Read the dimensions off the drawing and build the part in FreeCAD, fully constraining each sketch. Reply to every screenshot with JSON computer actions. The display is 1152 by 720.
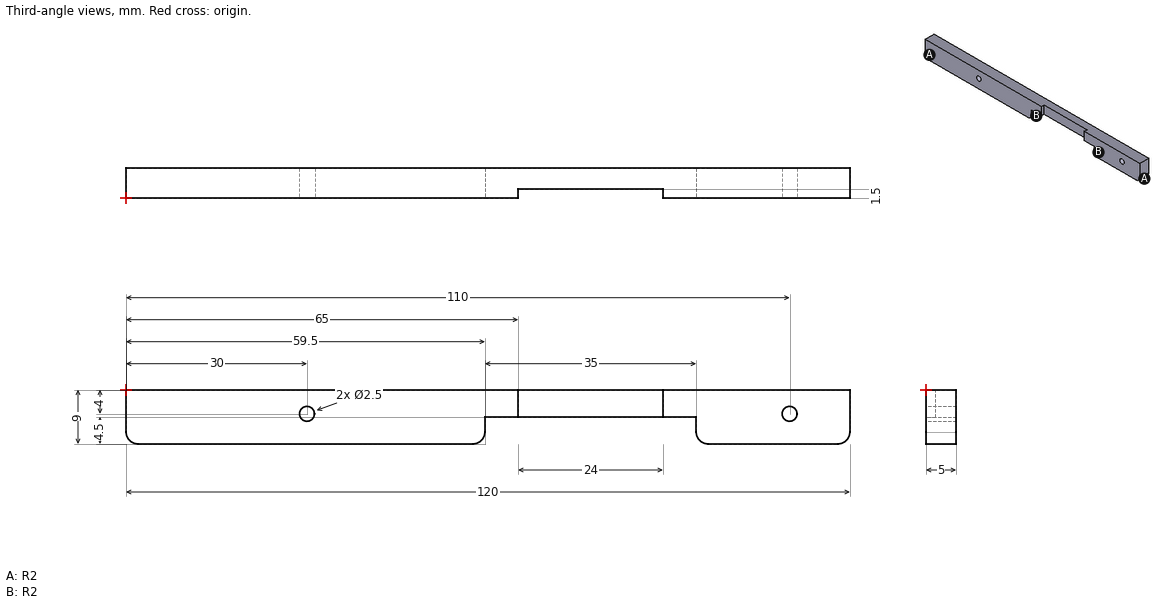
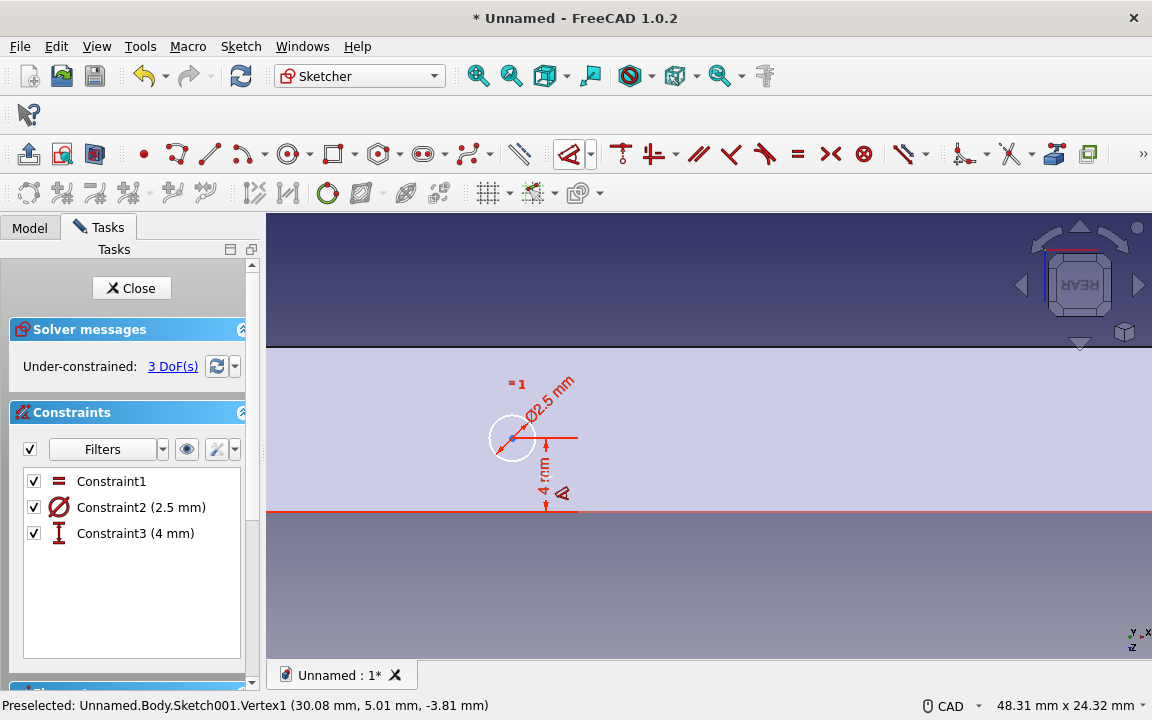
{"action": "scroll", "coordinate": [529, 427], "scroll_direction": "down", "scroll_amount": 7}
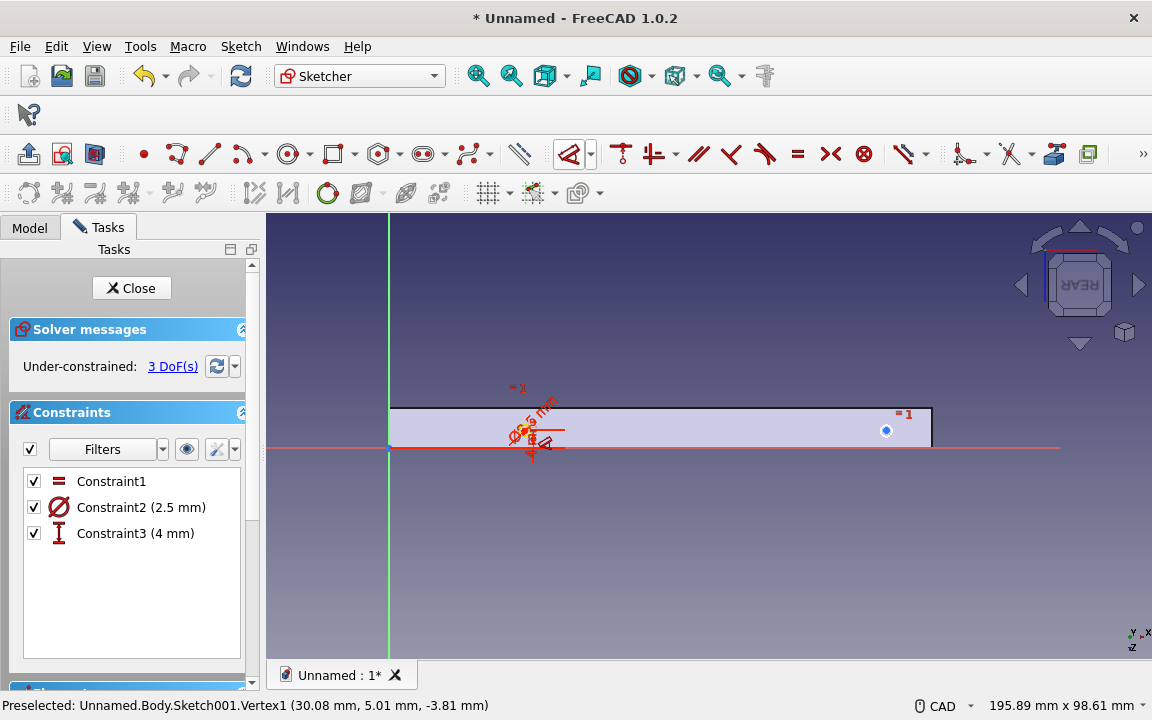
{"action": "scroll", "coordinate": [886, 431], "scroll_direction": "up", "scroll_amount": 4}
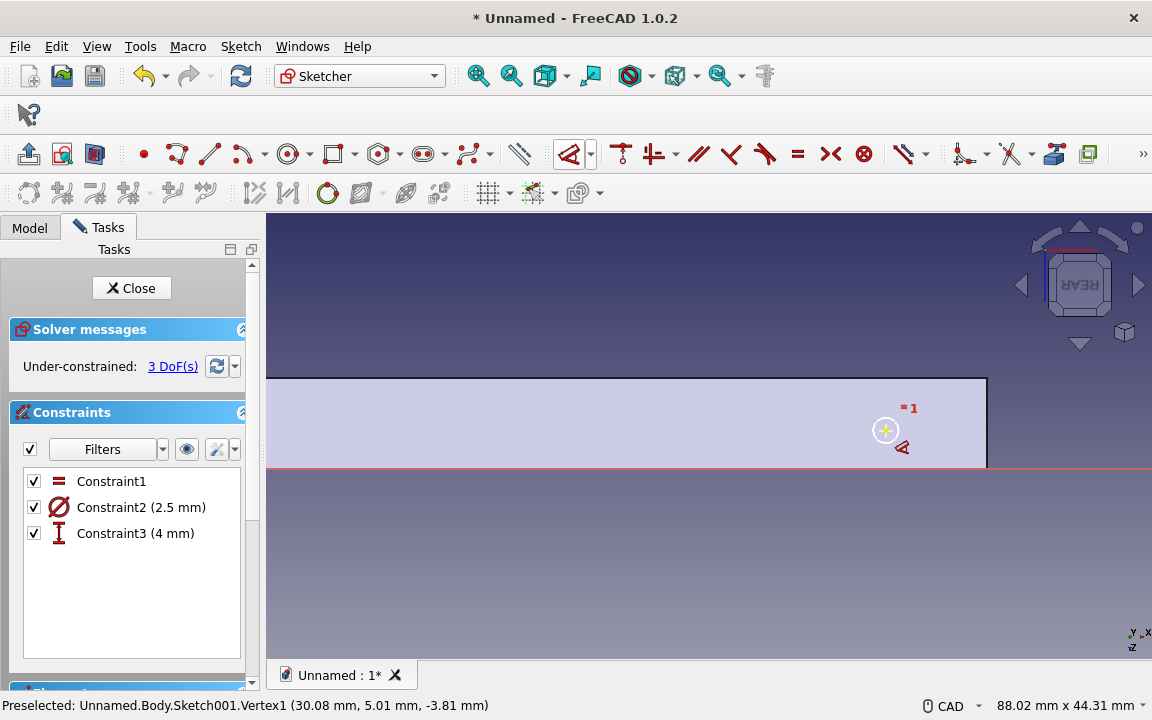
{"action": "left_click", "coordinate": [886, 430]}
{"action": "left_click", "coordinate": [920, 450]}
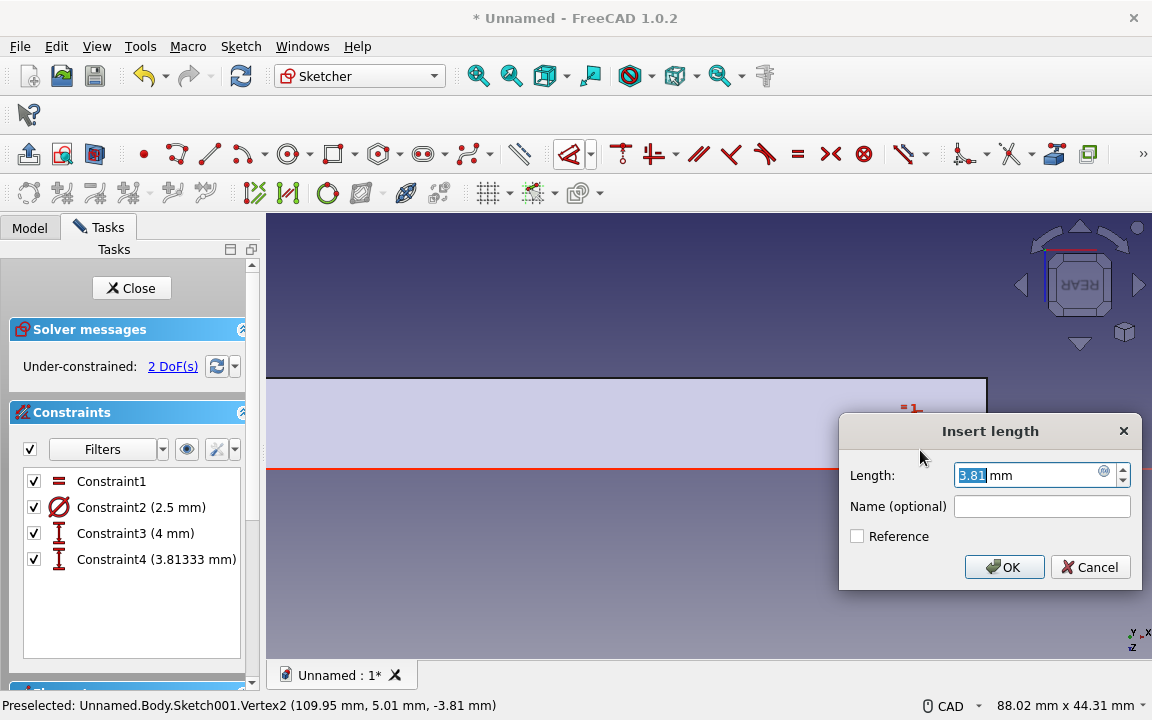
{"action": "type", "text": "4"}
{"action": "key", "text": "Return"}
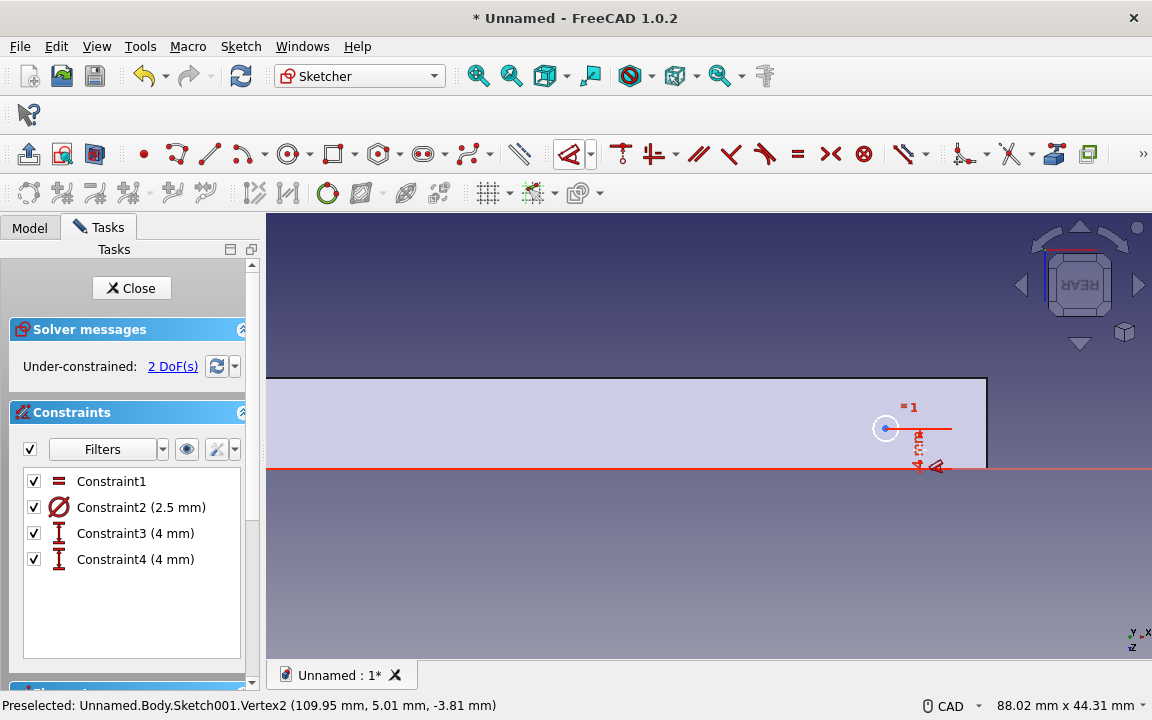
{"action": "scroll", "coordinate": [886, 431], "scroll_direction": "down", "scroll_amount": 4}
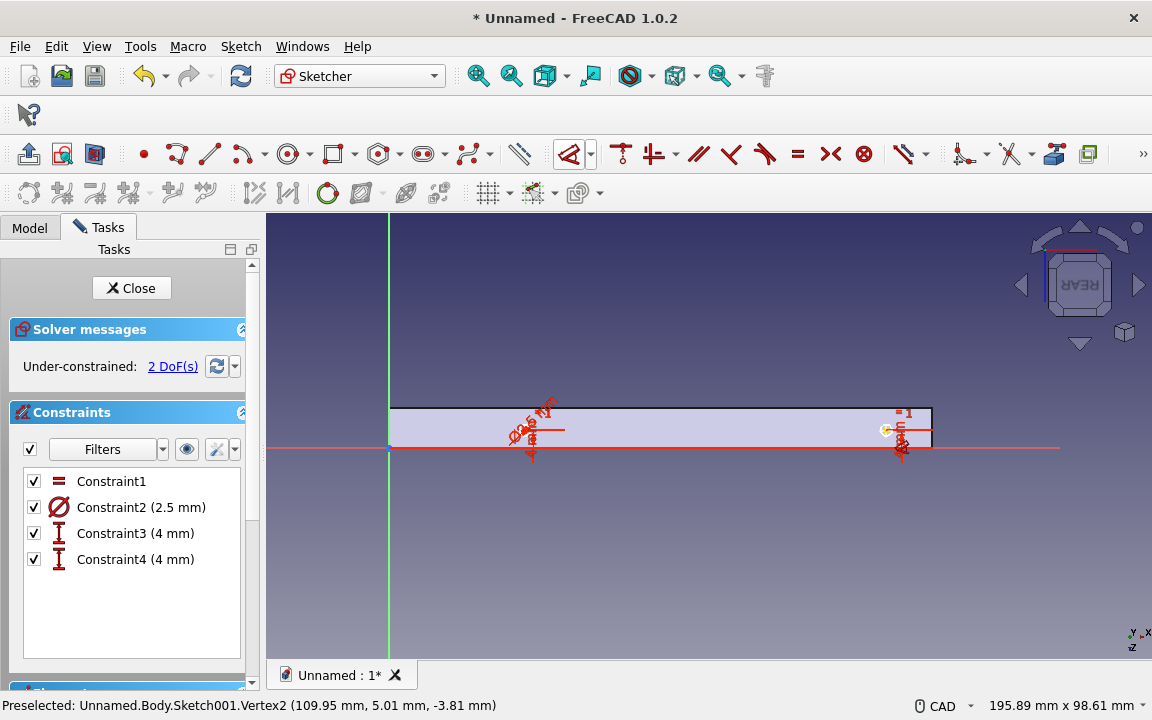
{"action": "left_click", "coordinate": [525, 430]}
{"action": "left_click", "coordinate": [457, 482]}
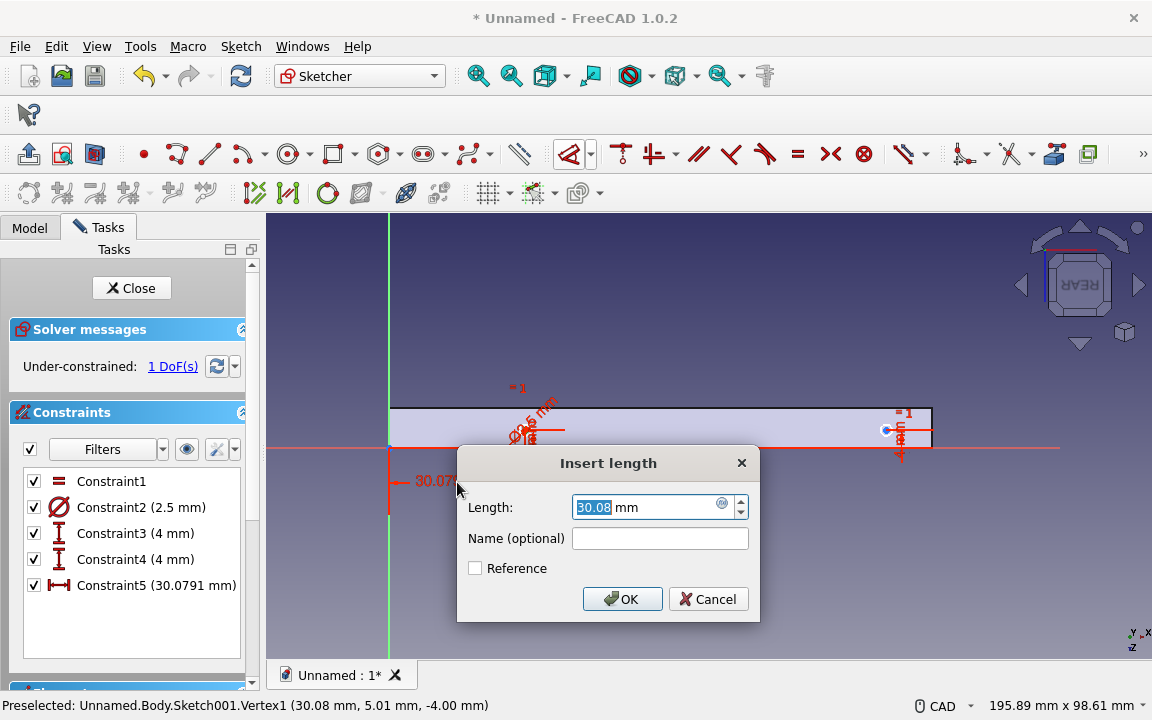
{"action": "type", "text": "30"}
{"action": "key", "text": "Return"}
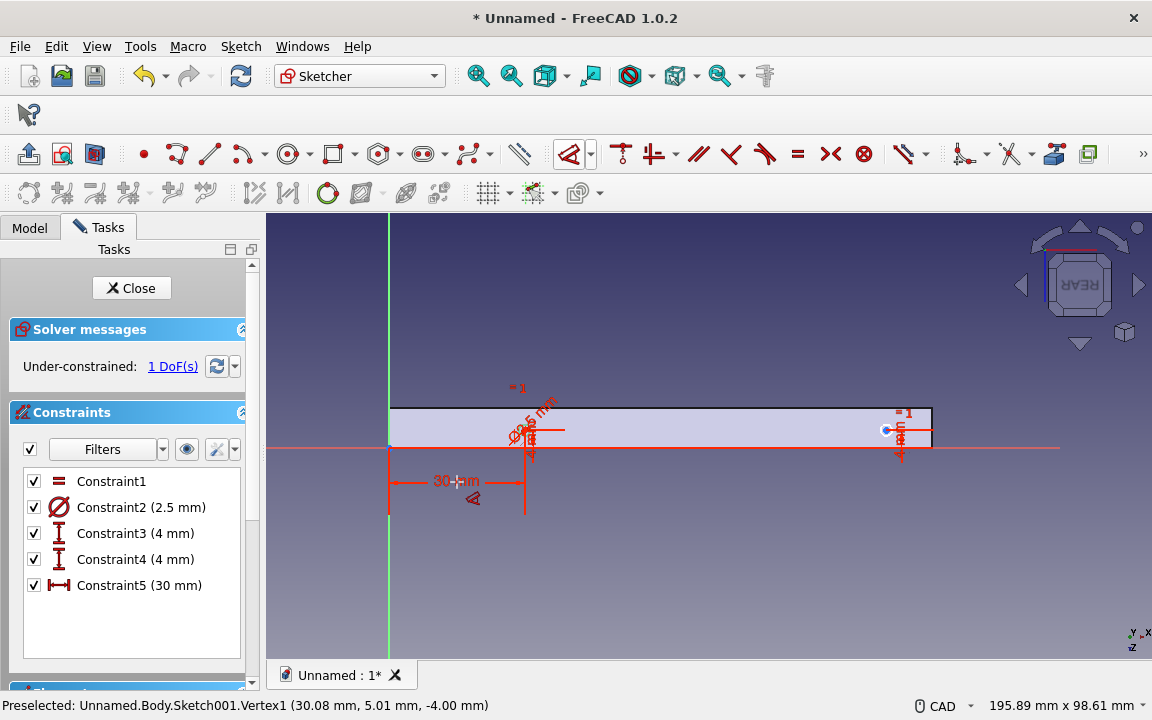
{"action": "left_click", "coordinate": [886, 430]}
{"action": "left_click", "coordinate": [638, 482]}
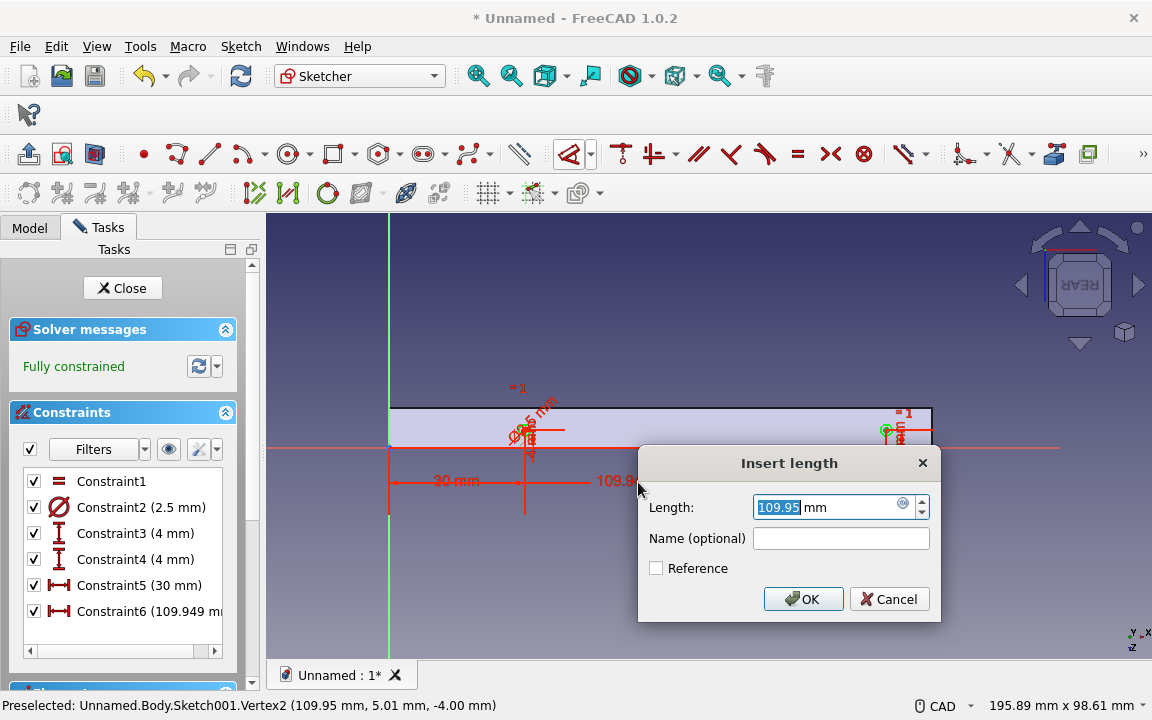
{"action": "type", "text": "110"}
{"action": "key", "text": "Return"}
{"action": "key", "text": "Escape"}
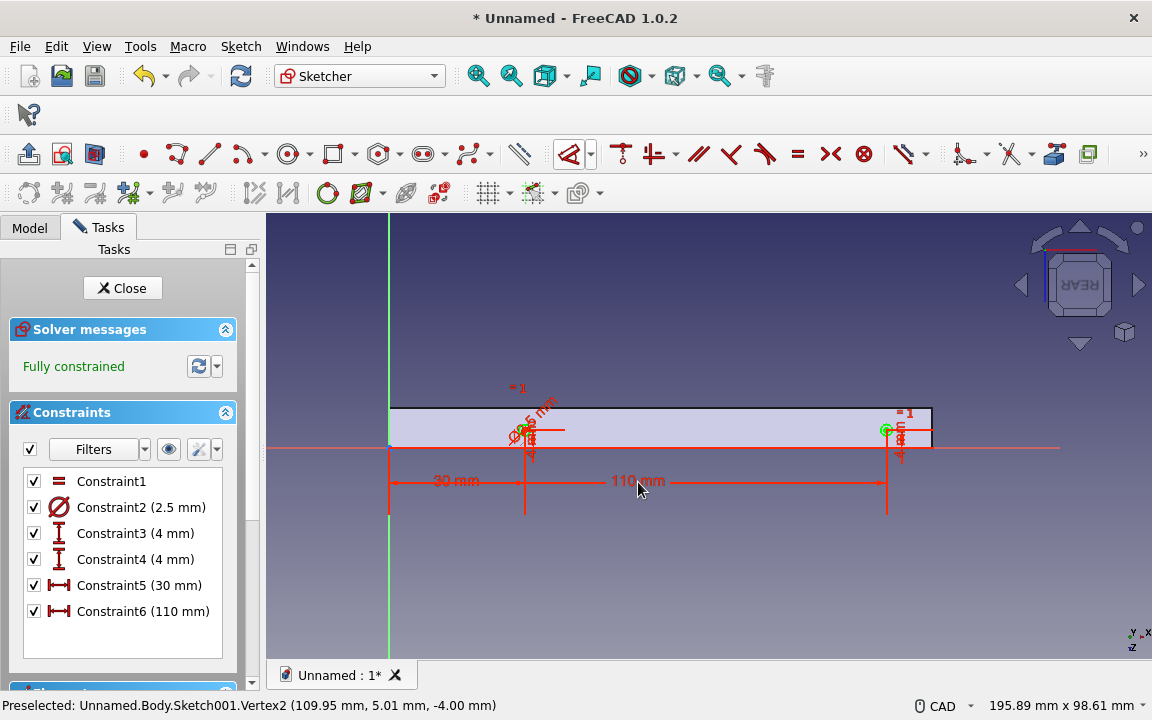
{"action": "left_click", "coordinate": [123, 288]}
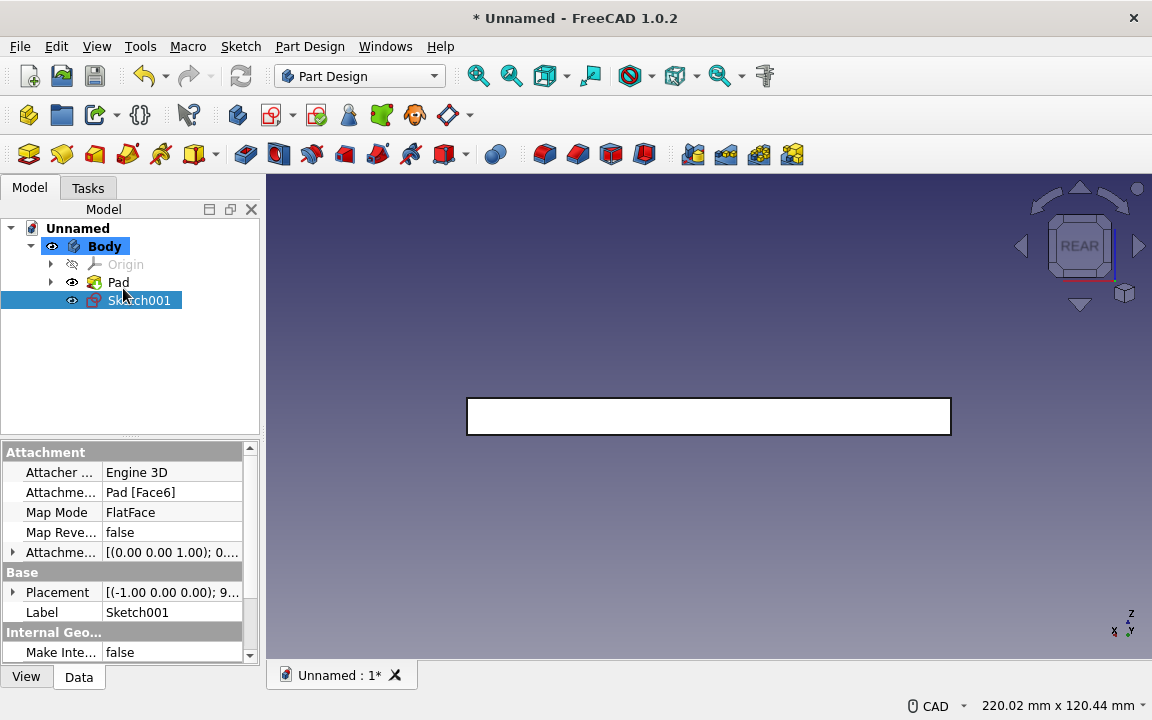
{"action": "left_click", "coordinate": [246, 154]}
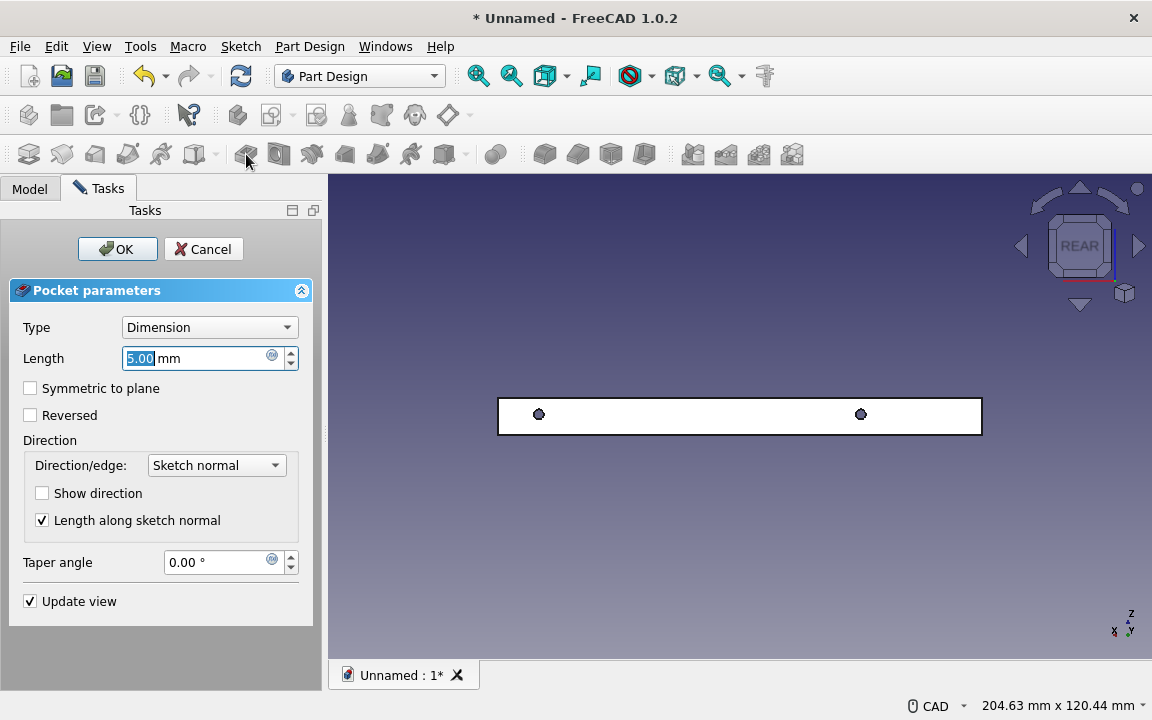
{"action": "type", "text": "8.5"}
{"action": "key", "text": "Tab"}